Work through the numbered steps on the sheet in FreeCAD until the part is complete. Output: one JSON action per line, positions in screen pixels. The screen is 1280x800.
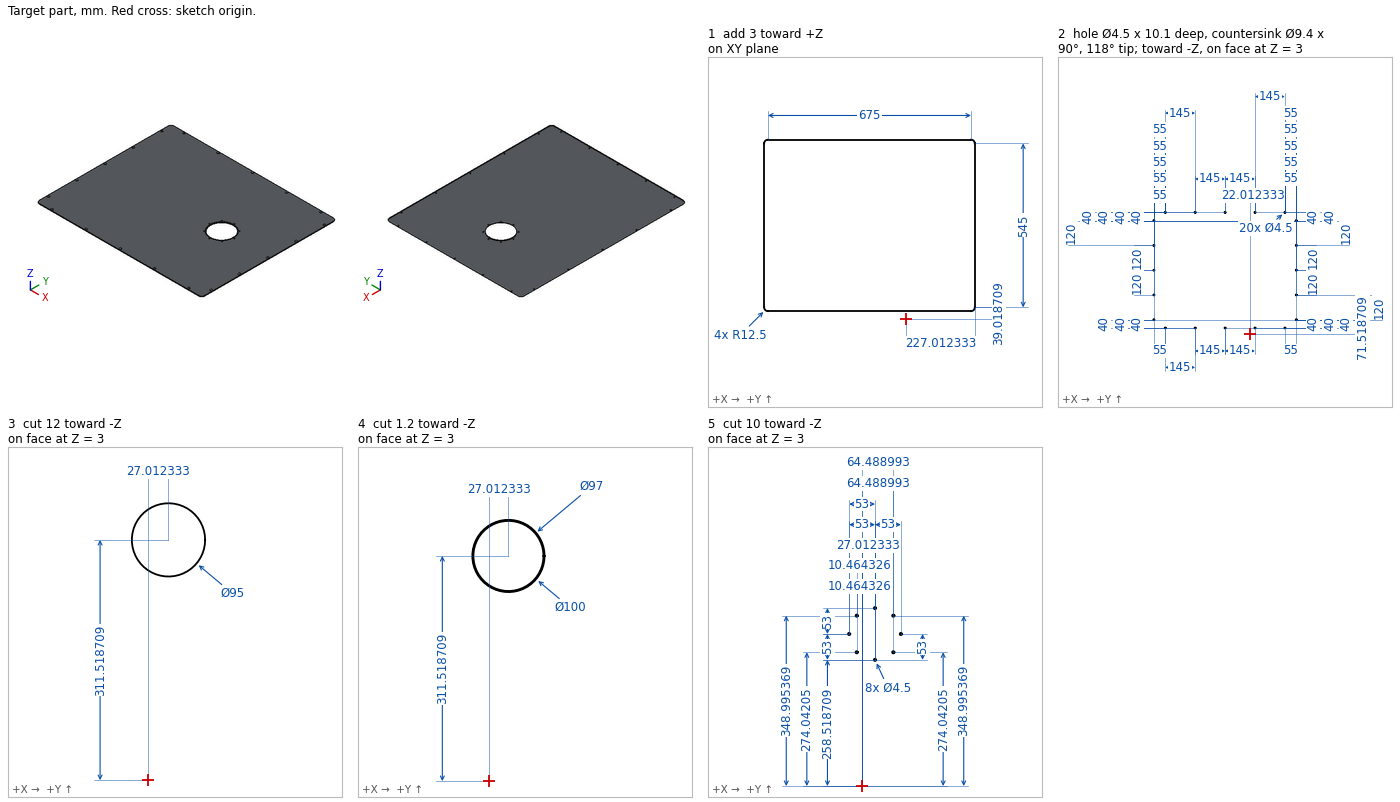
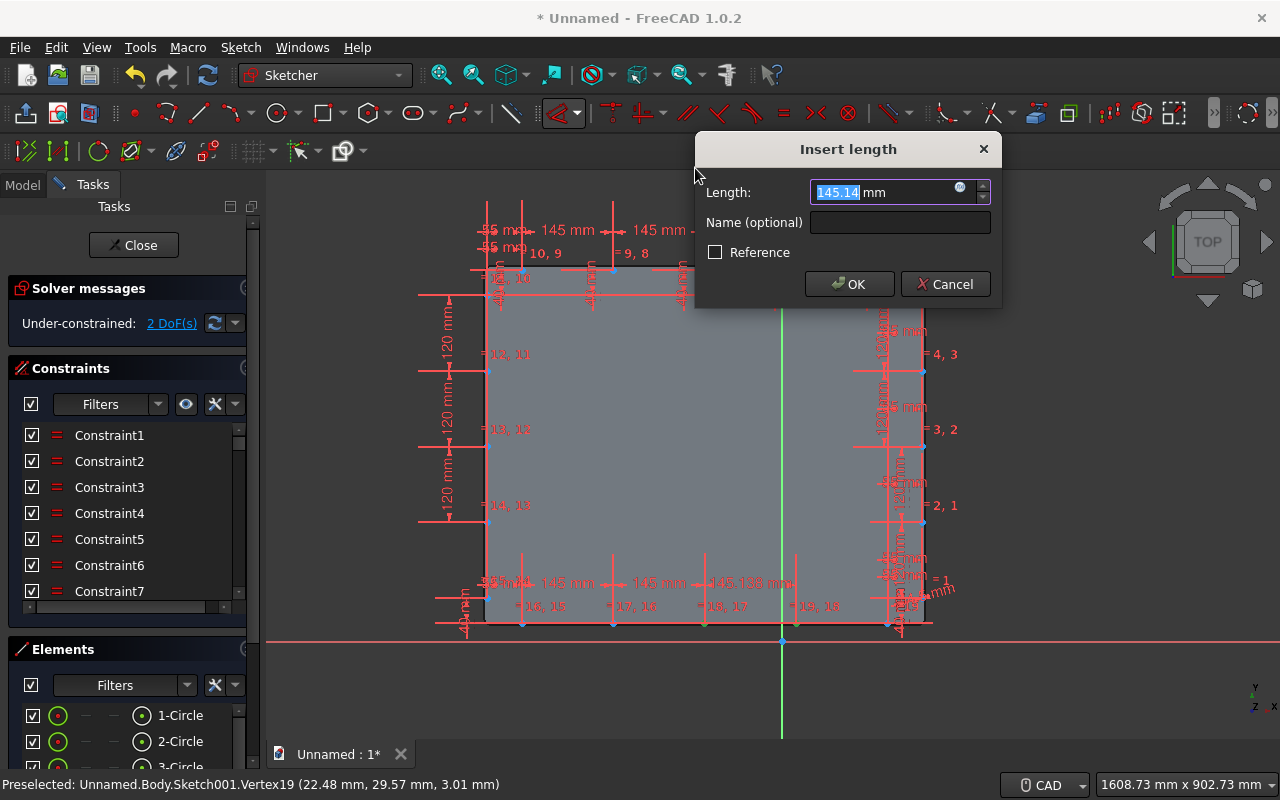
{"action": "type", "text": "145"}
{"action": "key", "text": "Return"}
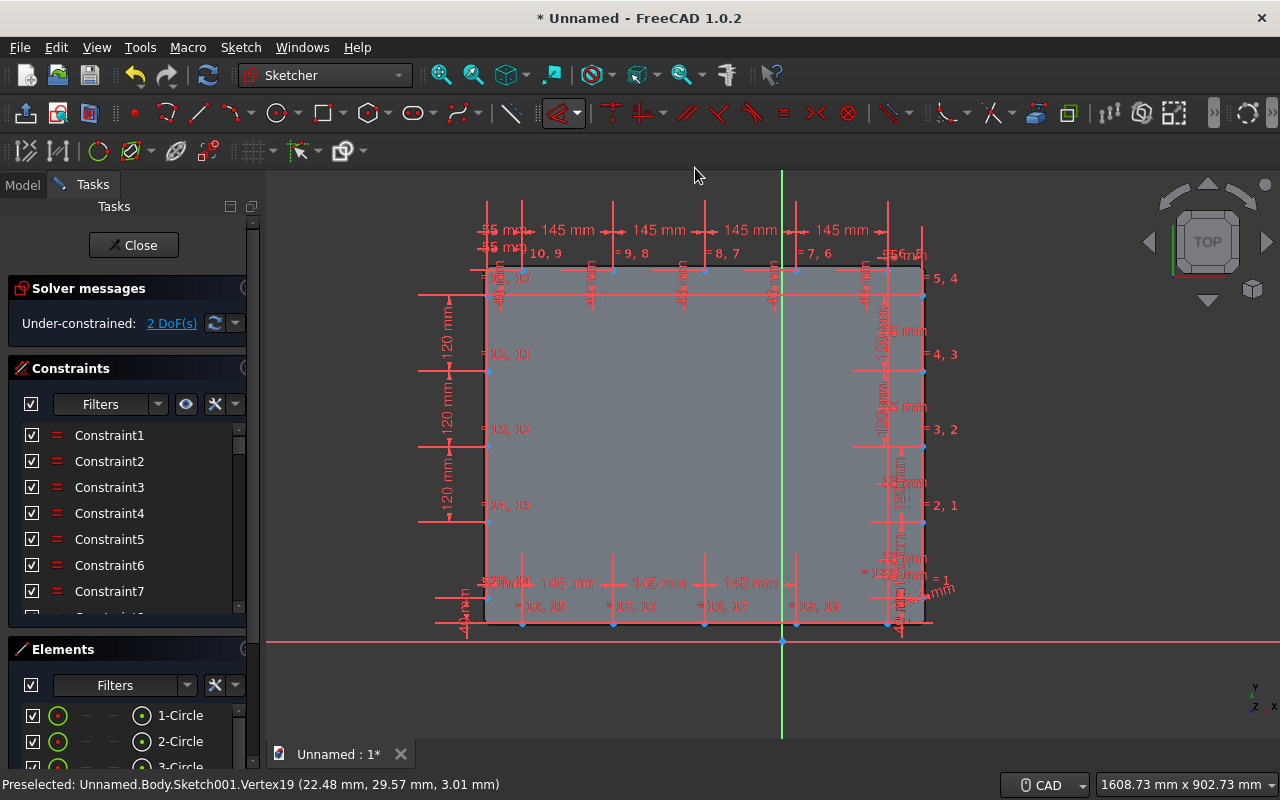
{"action": "left_click", "coordinate": [922, 598]}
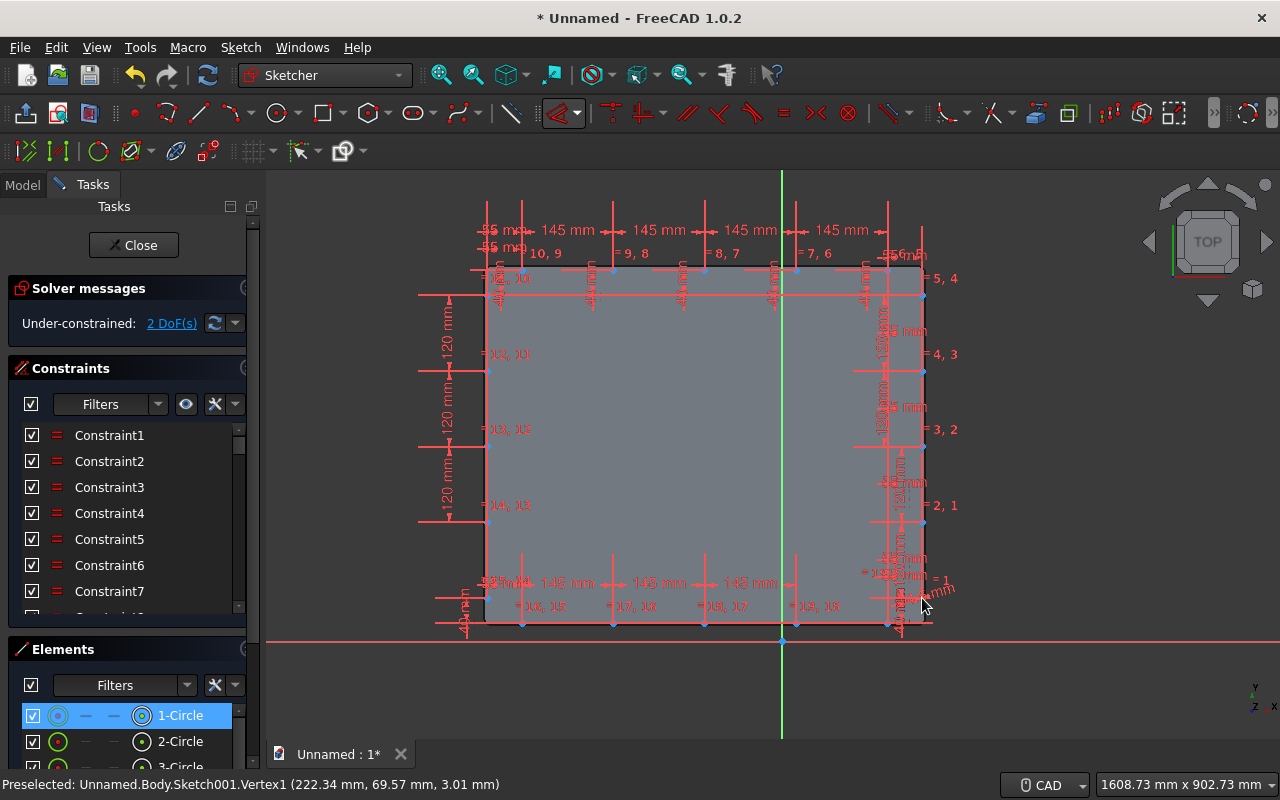
{"action": "key", "text": "i"}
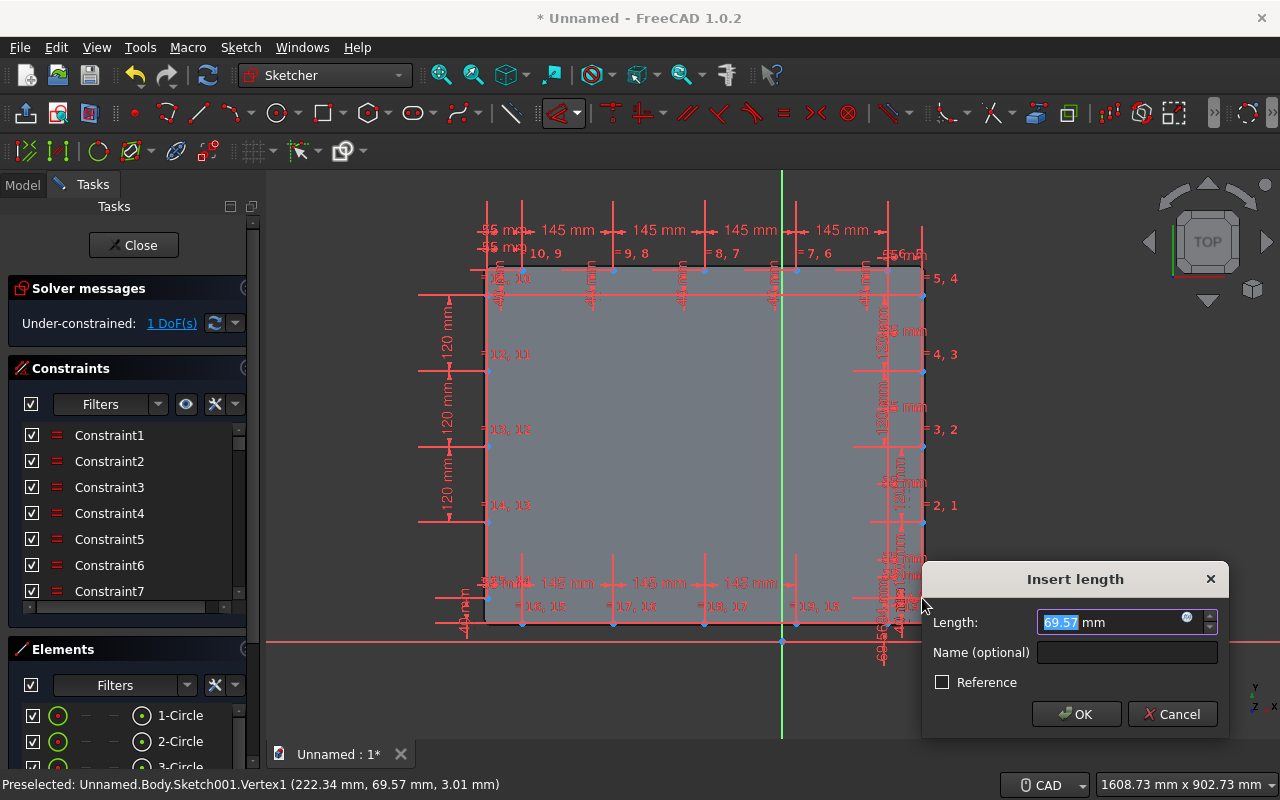
{"action": "type", "text": "71.518709"}
{"action": "key", "text": "Return"}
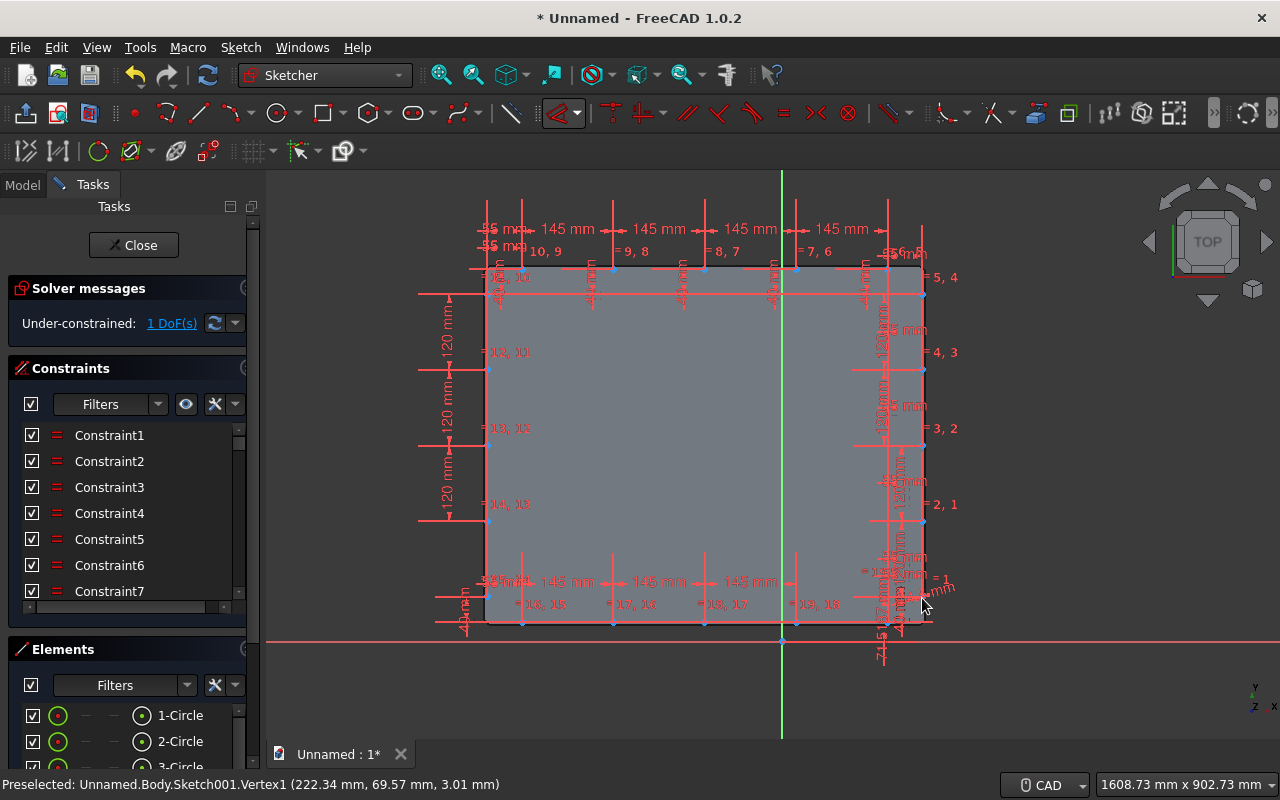
{"action": "scroll", "coordinate": [796, 269], "scroll_direction": "up", "scroll_amount": 6}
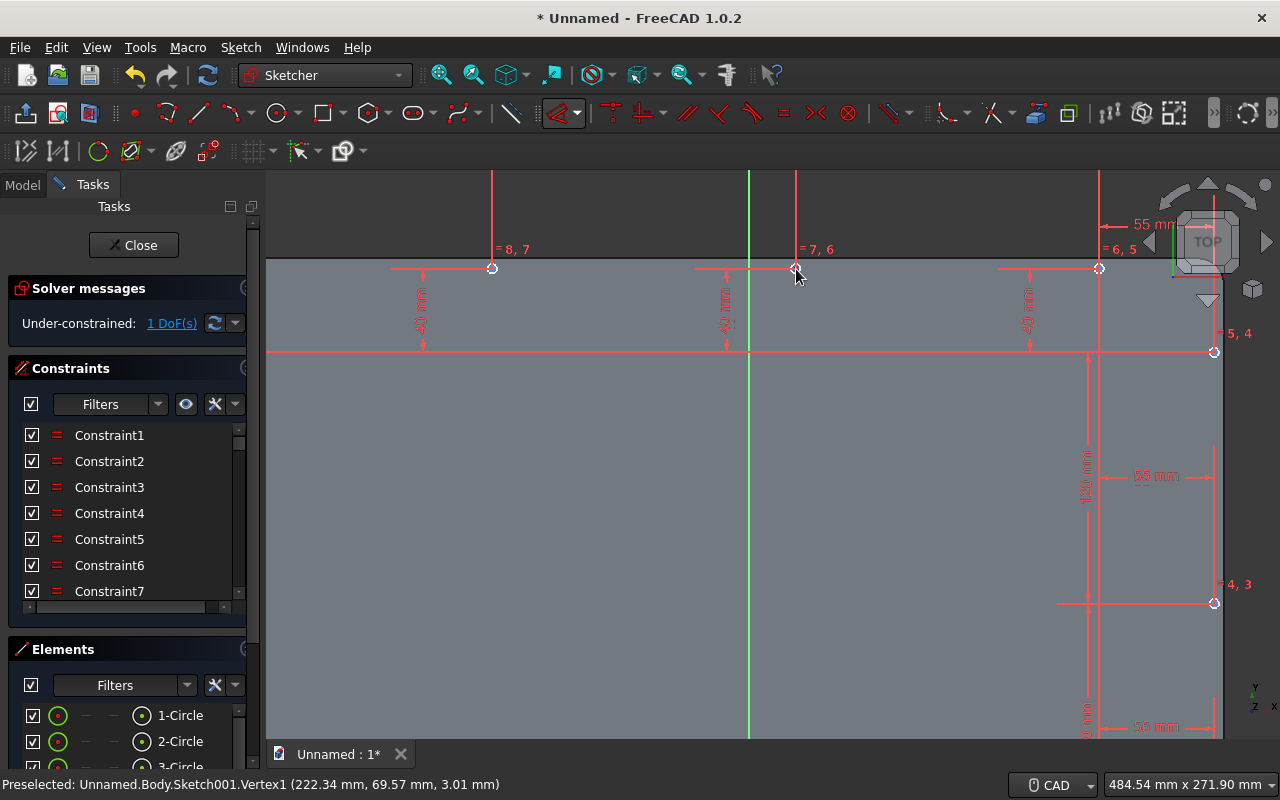
{"action": "left_click", "coordinate": [796, 269]}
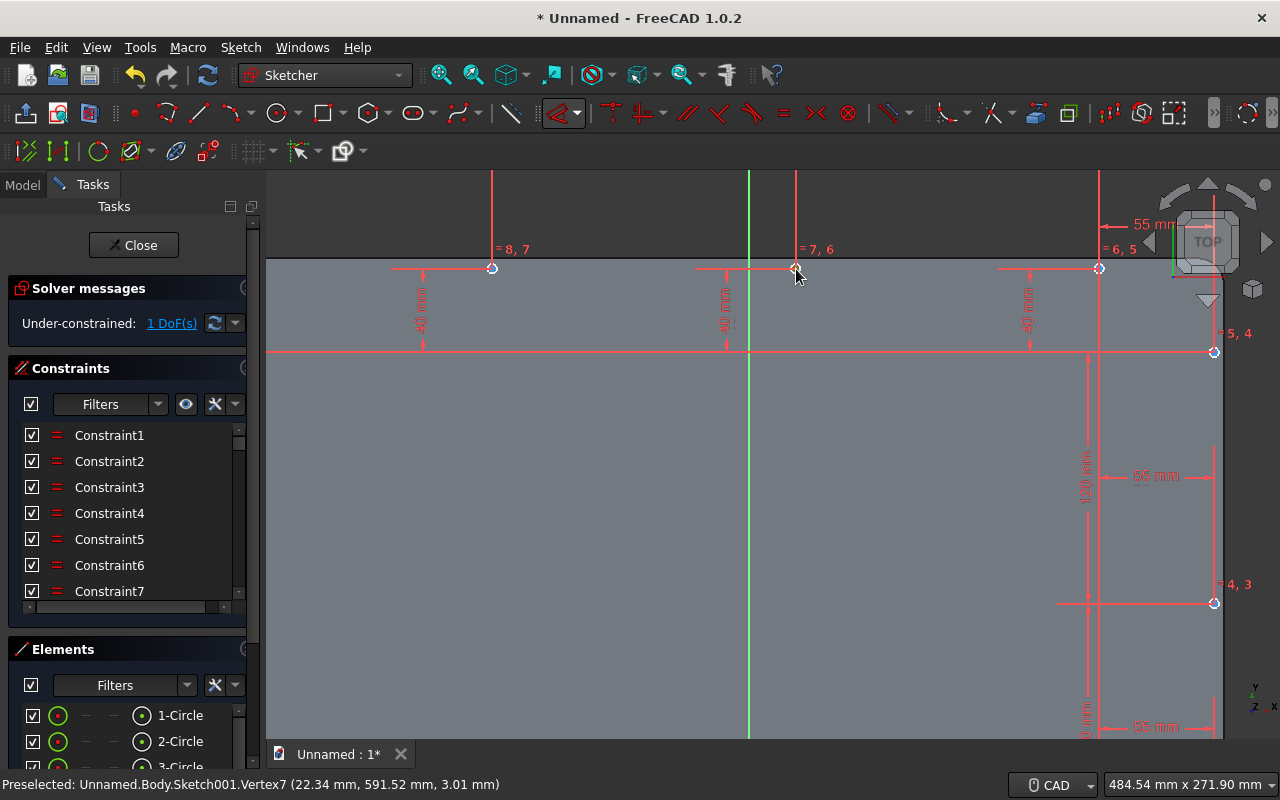
{"action": "left_click", "coordinate": [580, 114]}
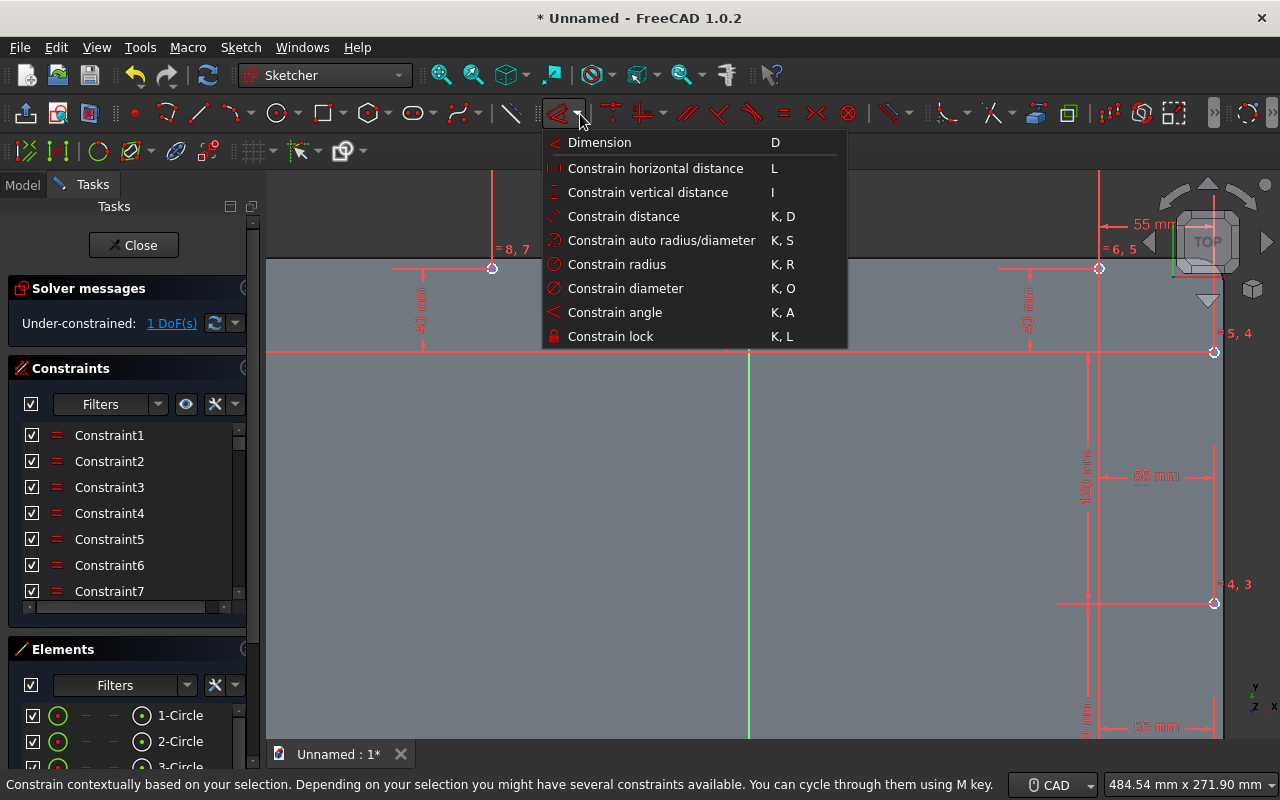
{"action": "left_click", "coordinate": [695, 168]}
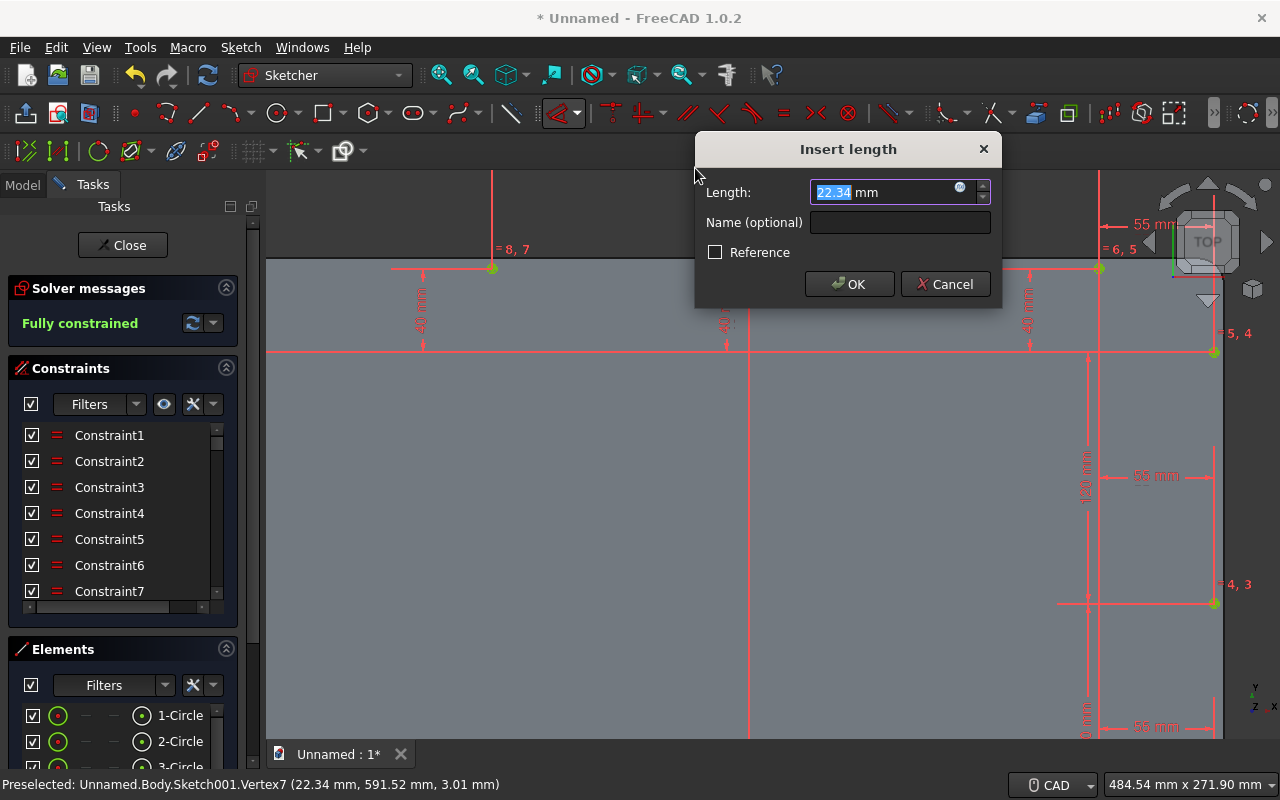
{"action": "type", "text": "22.012333"}
{"action": "key", "text": "Return"}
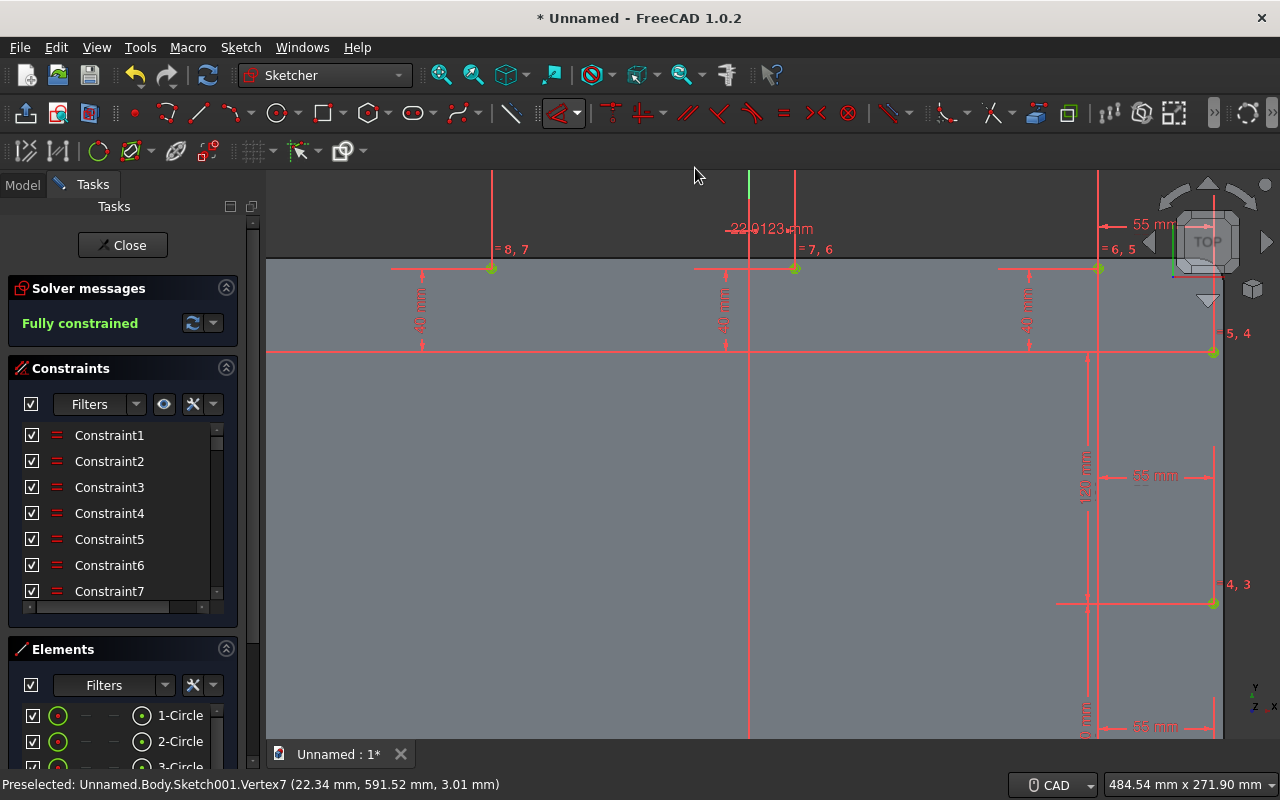
{"action": "left_click", "coordinate": [123, 245]}